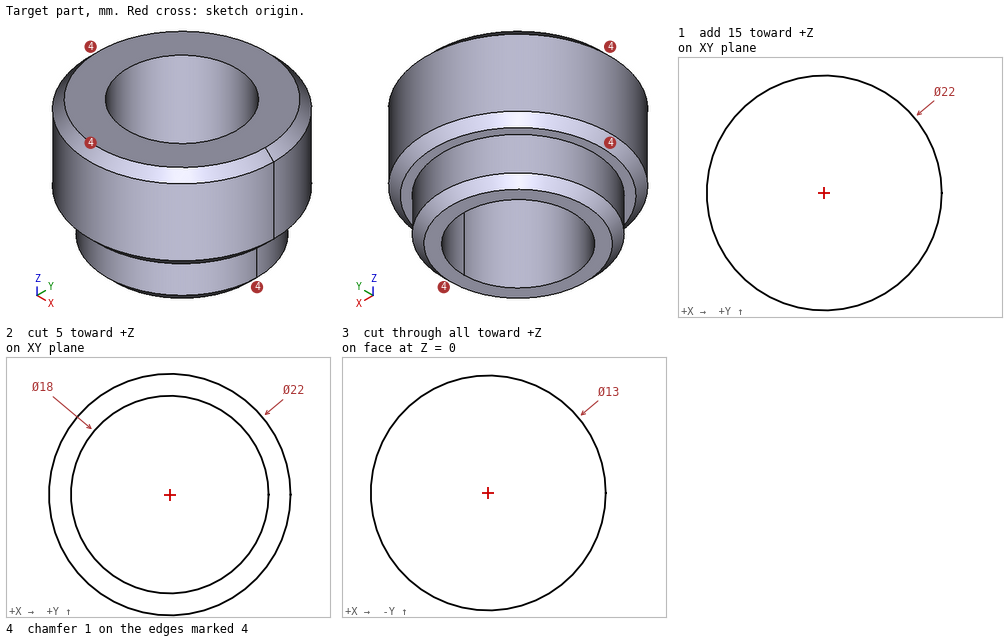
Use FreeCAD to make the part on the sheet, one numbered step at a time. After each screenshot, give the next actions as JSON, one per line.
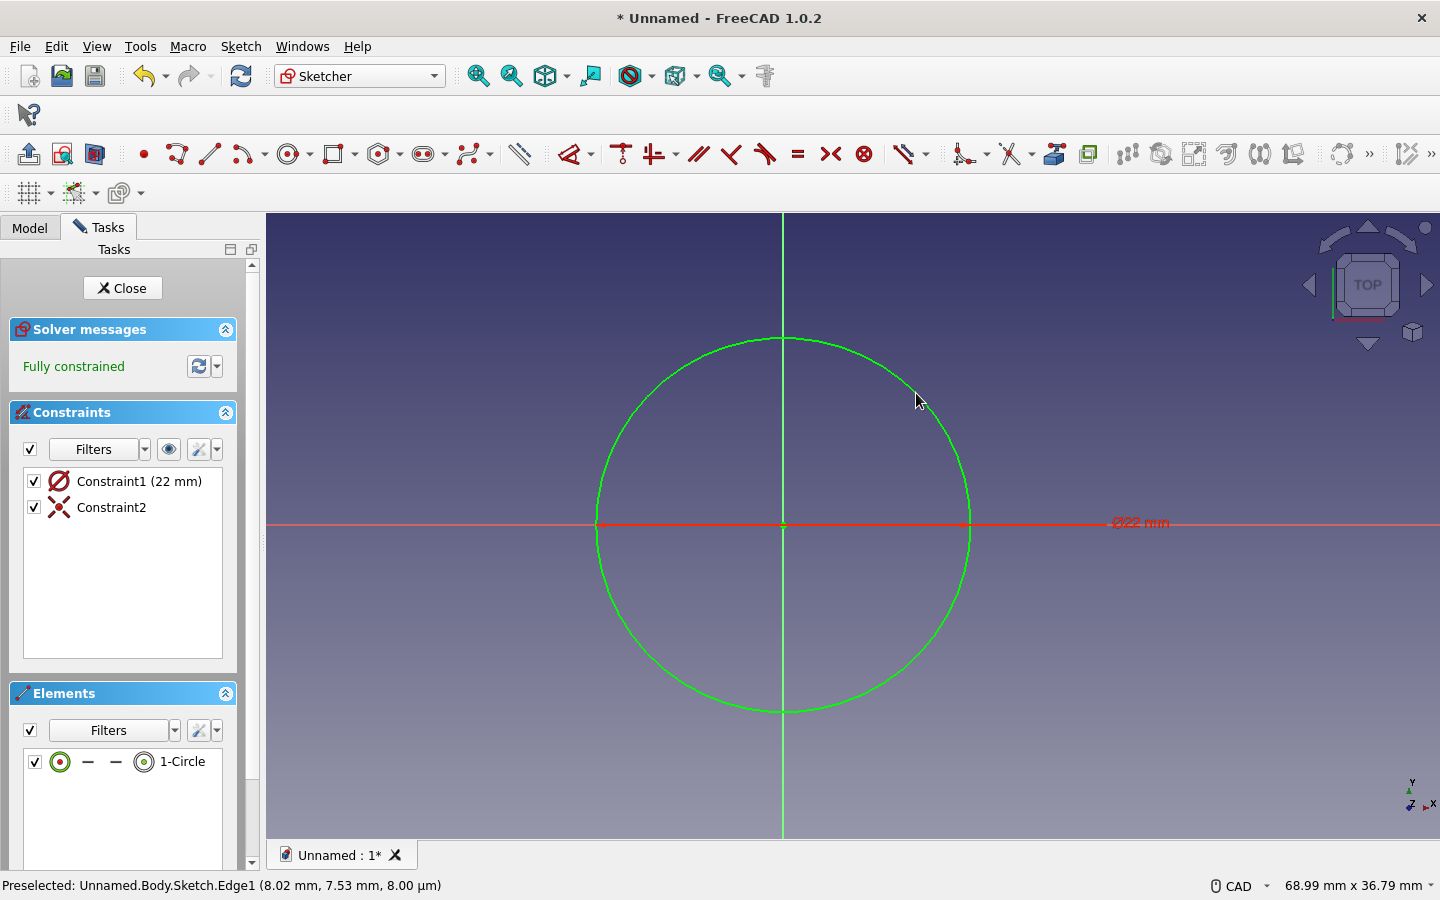
{"action": "left_click", "coordinate": [123, 288]}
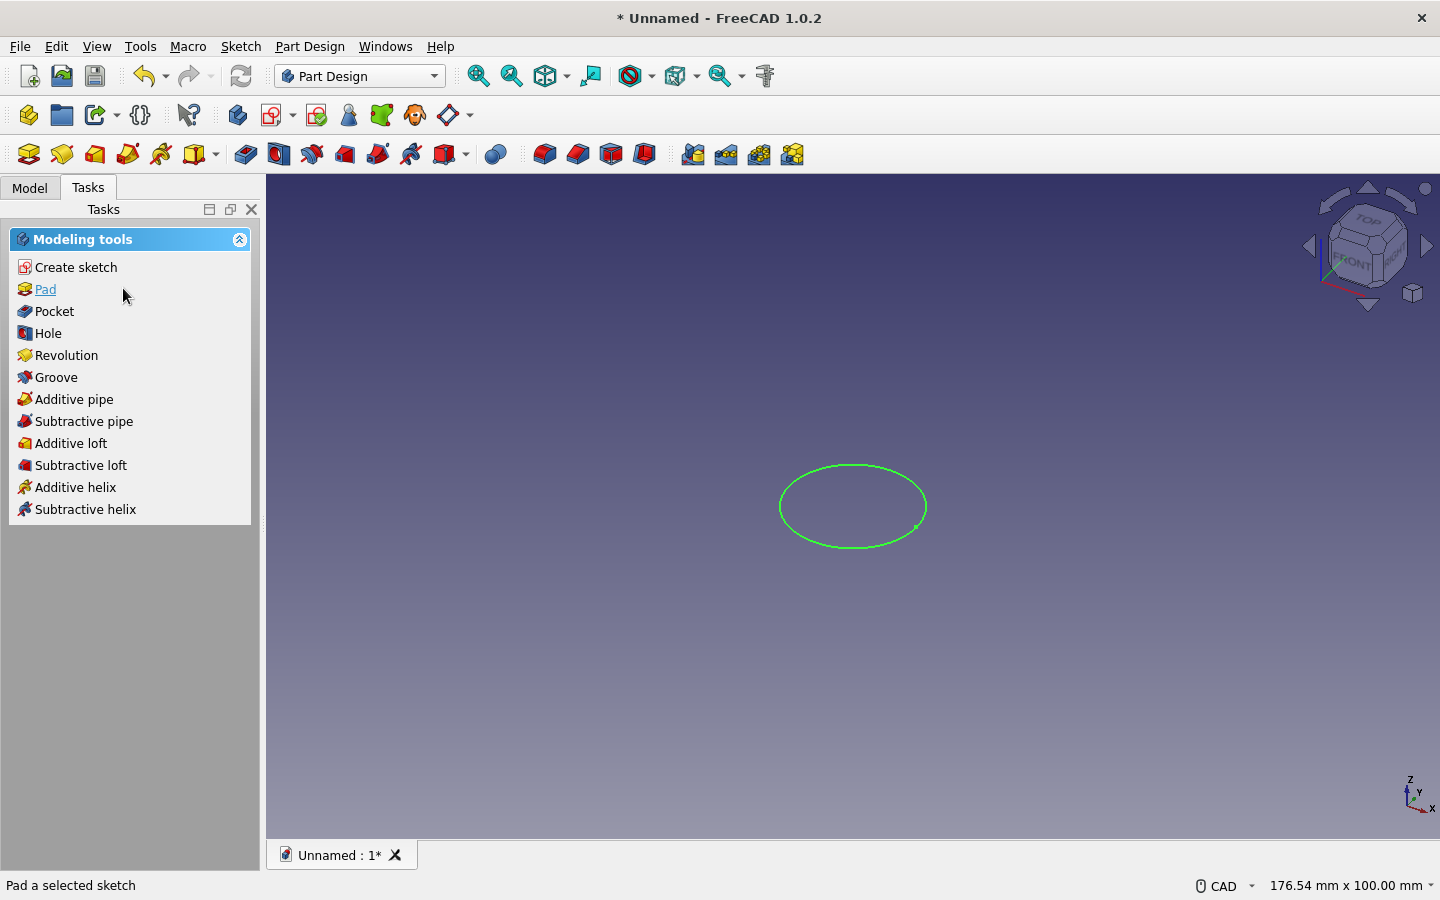
{"action": "left_click", "coordinate": [29, 154]}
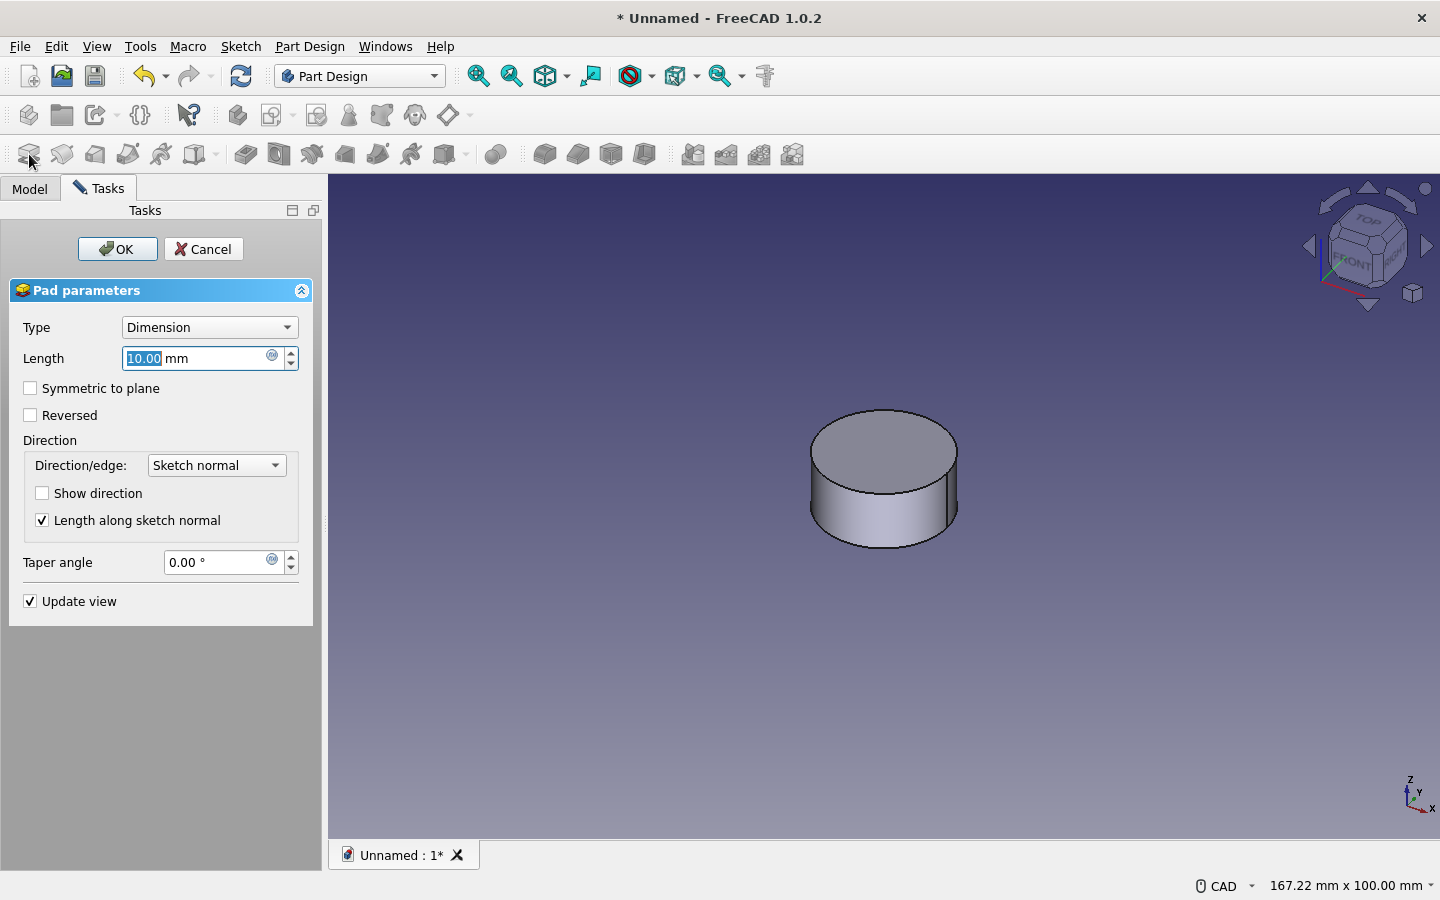
{"action": "type", "text": "15"}
{"action": "key", "text": "Tab"}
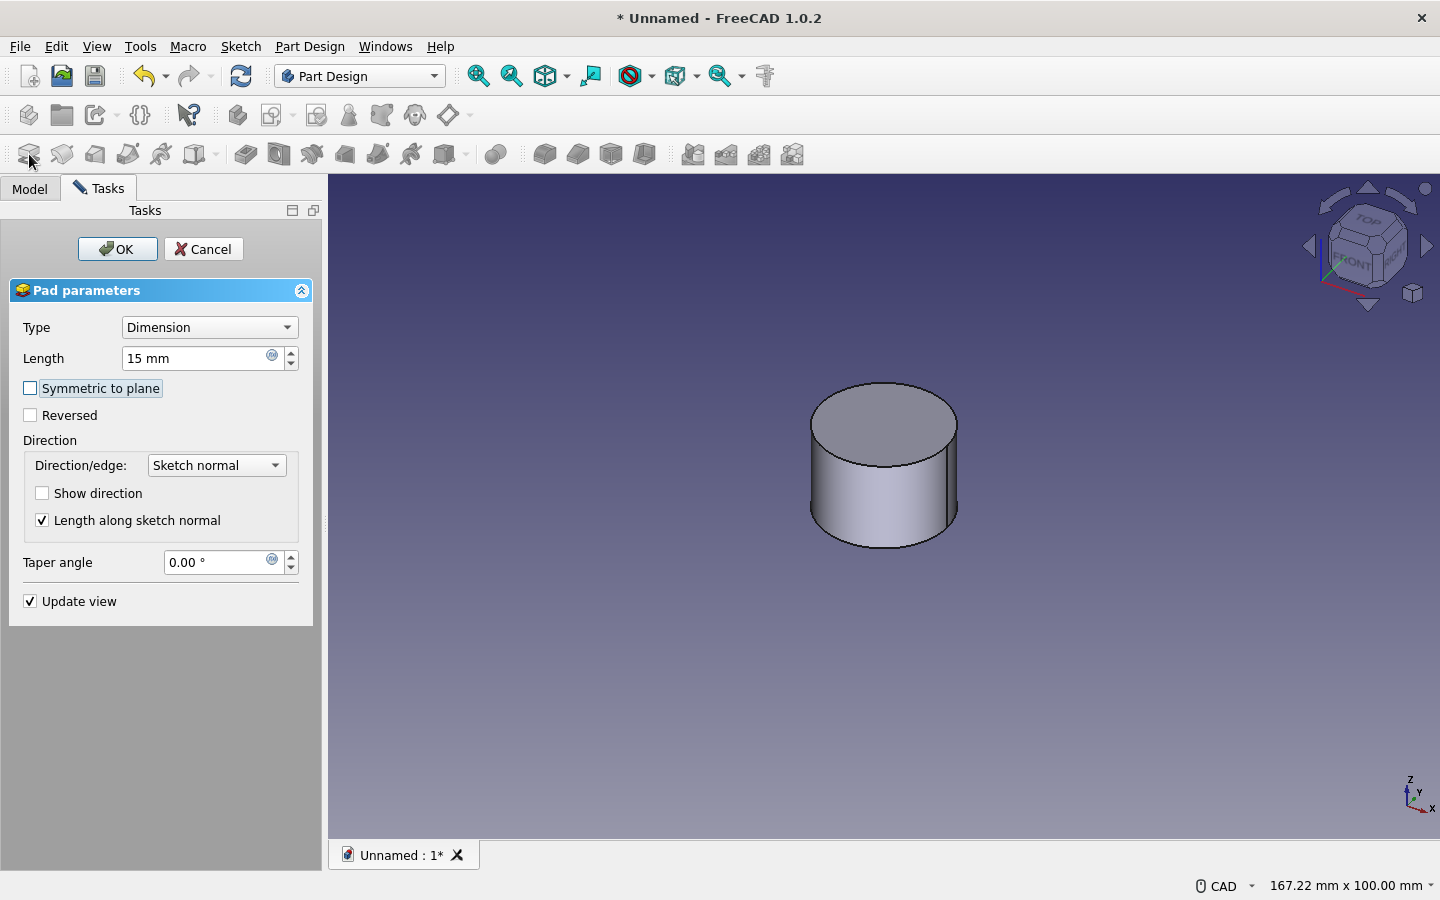
{"action": "left_click", "coordinate": [118, 249]}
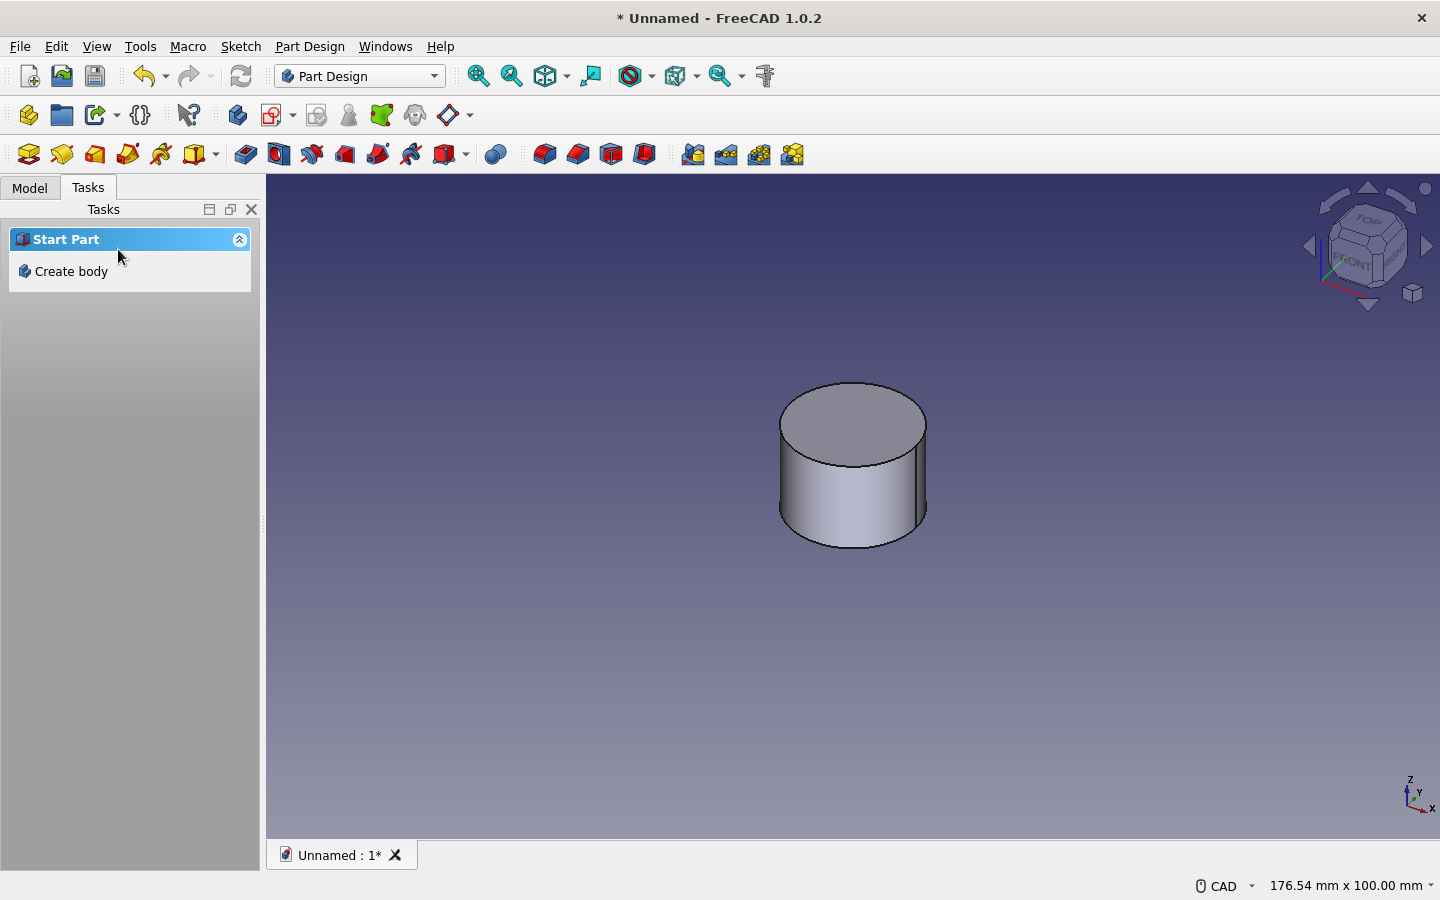
{"action": "left_click", "coordinate": [479, 76]}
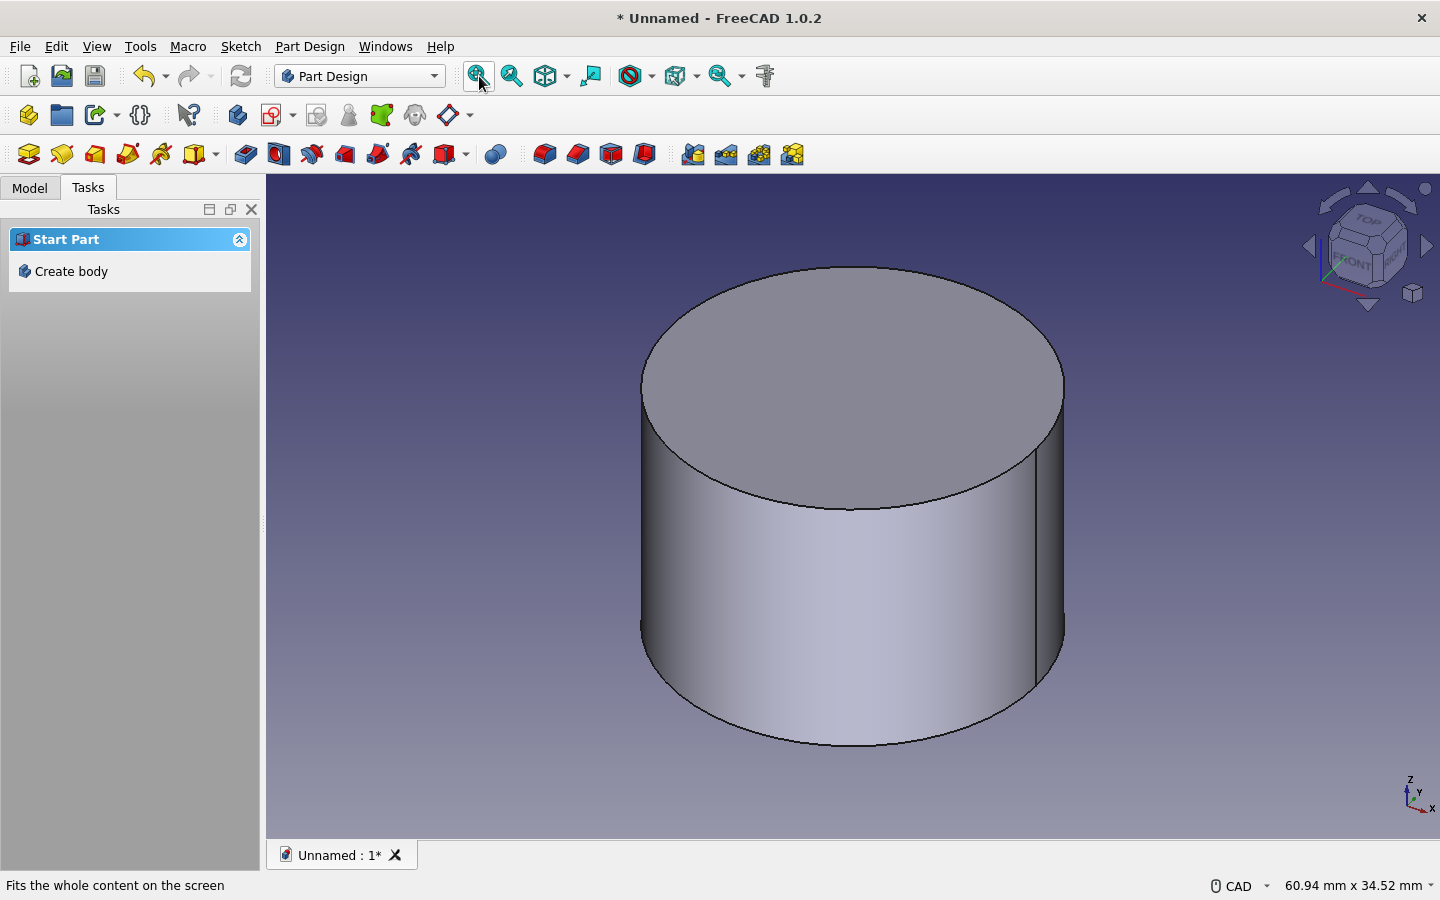
{"action": "left_click", "coordinate": [270, 116]}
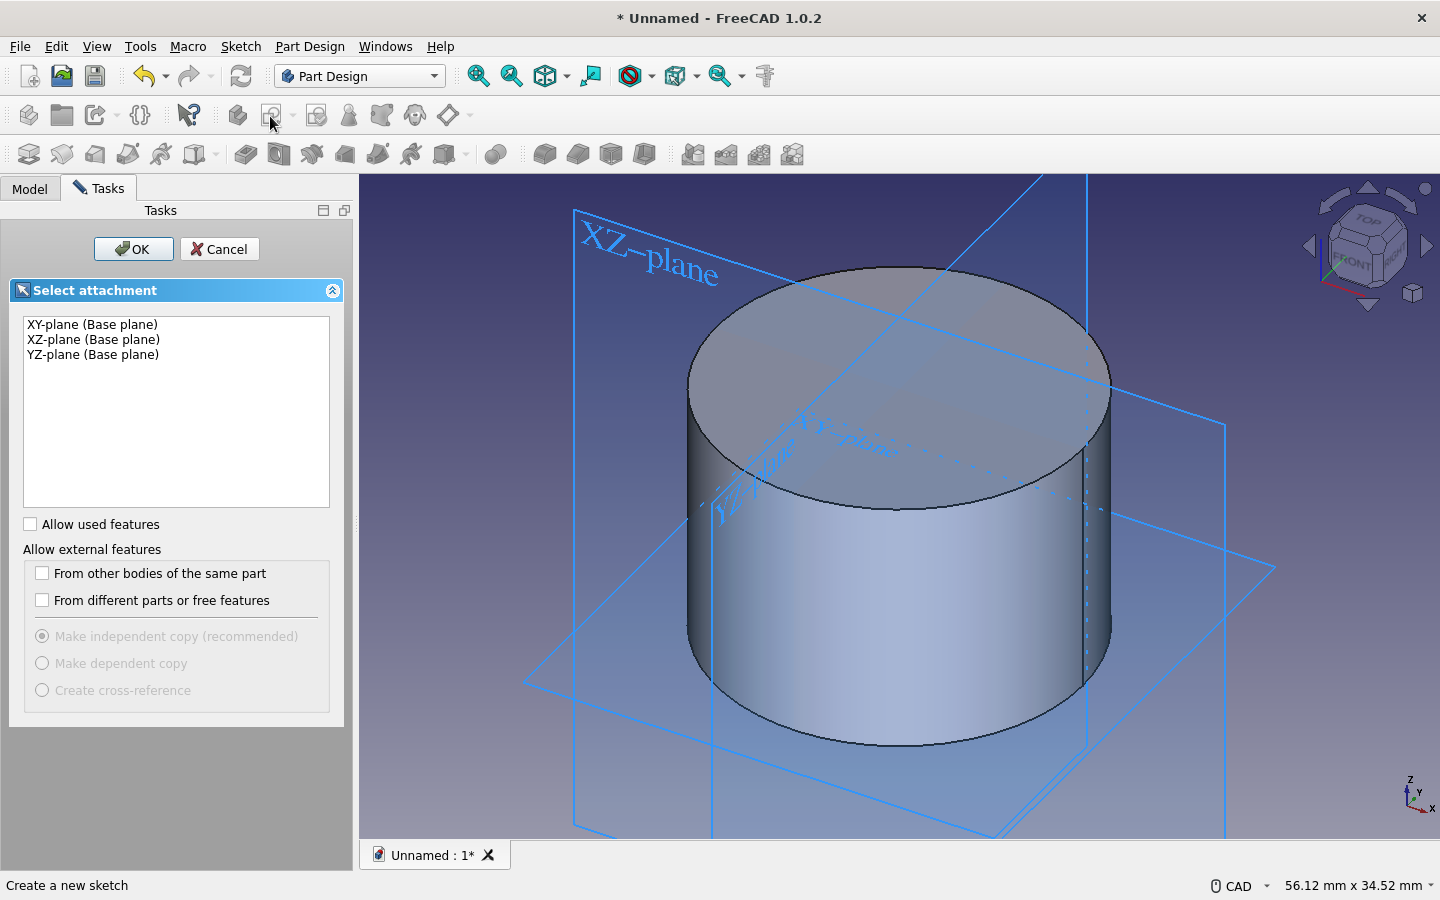
{"action": "left_click", "coordinate": [84, 324]}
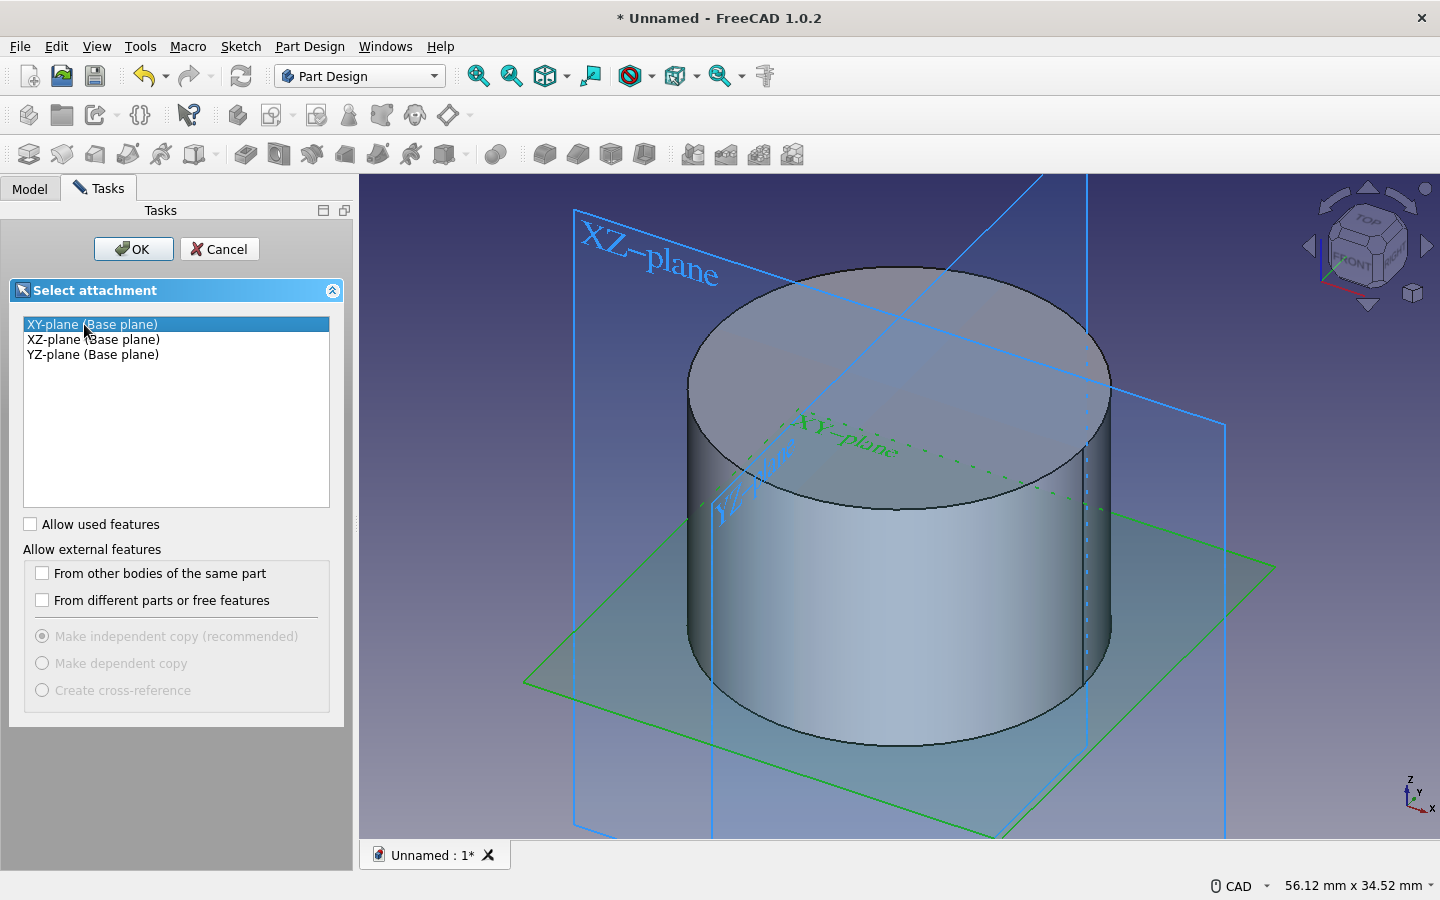
{"action": "left_click", "coordinate": [134, 249]}